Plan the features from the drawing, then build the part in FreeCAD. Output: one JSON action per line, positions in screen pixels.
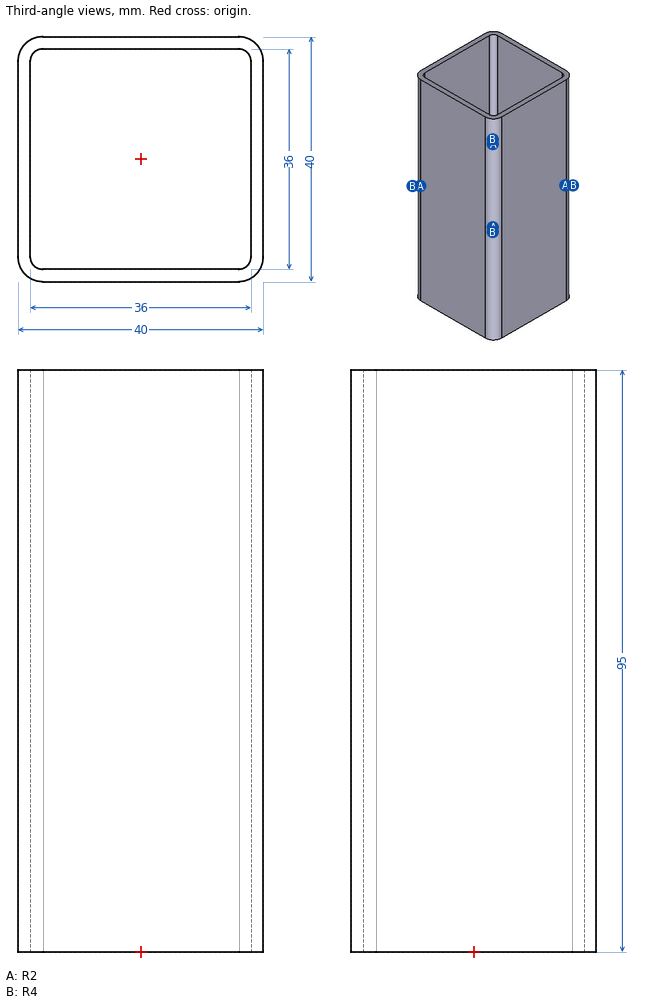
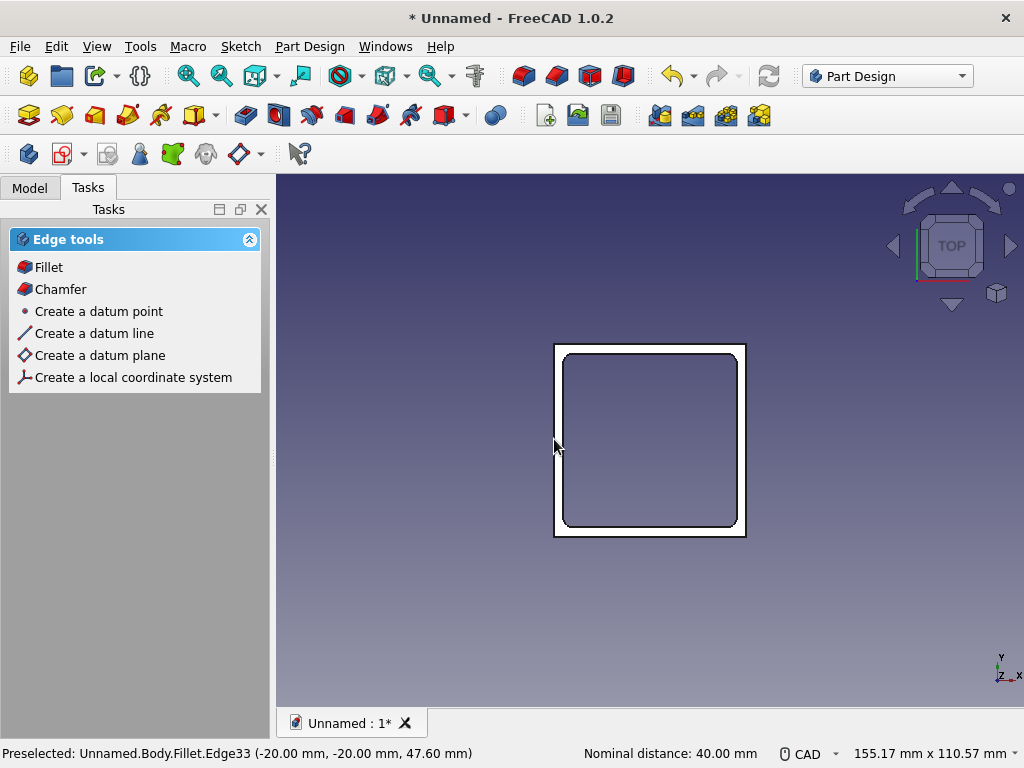
{"action": "key", "text": "v f"}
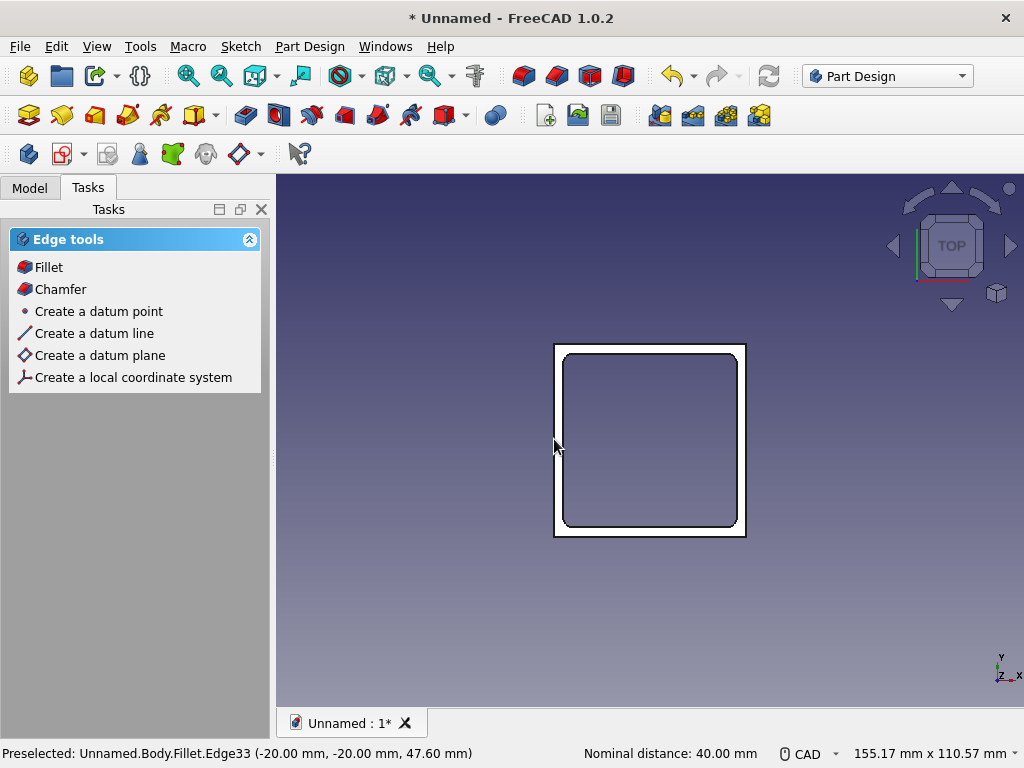
{"action": "key", "text": "1"}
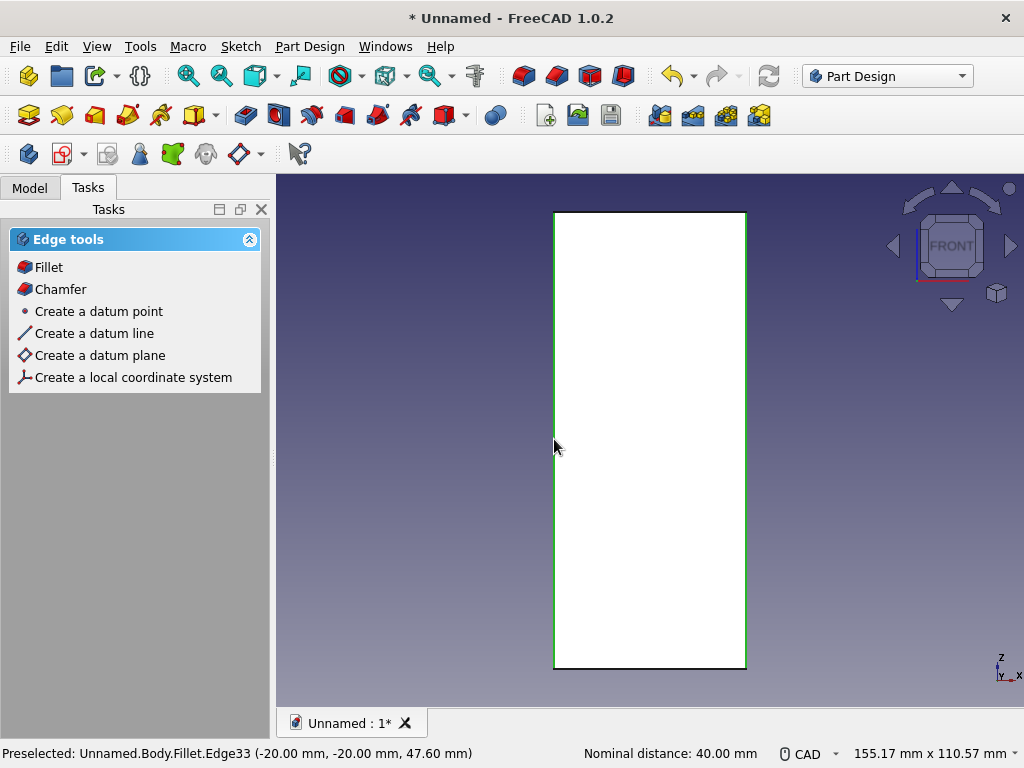
{"action": "key", "text": "3"}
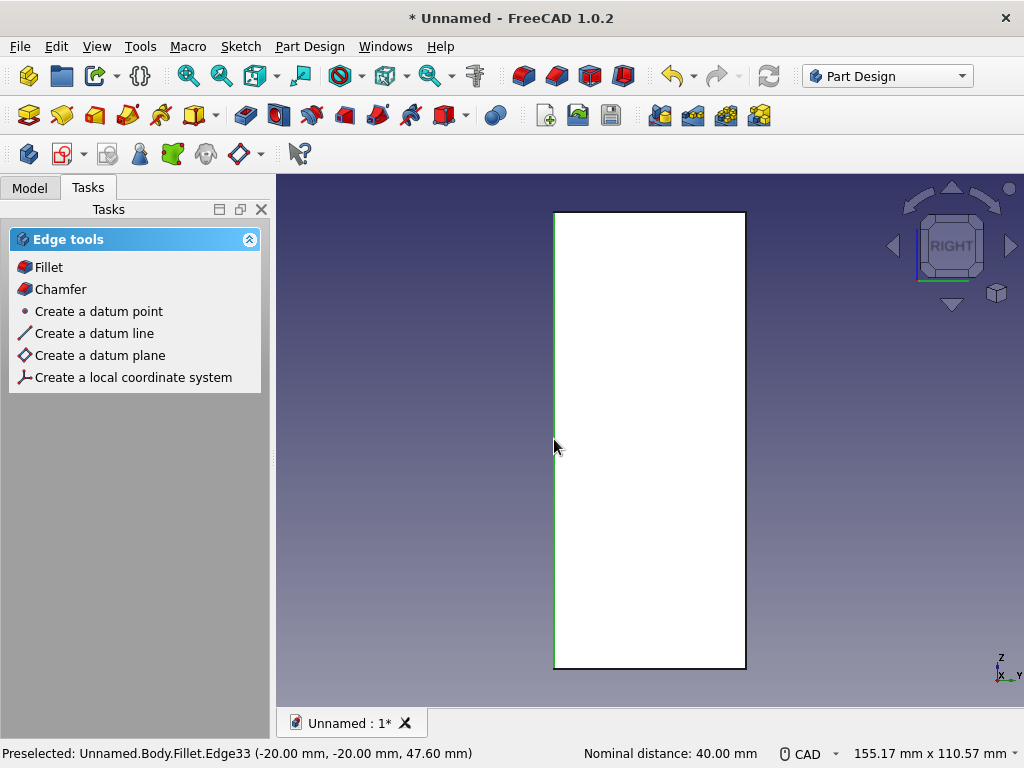
{"action": "left_click", "coordinate": [746, 439], "text": "ctrl"}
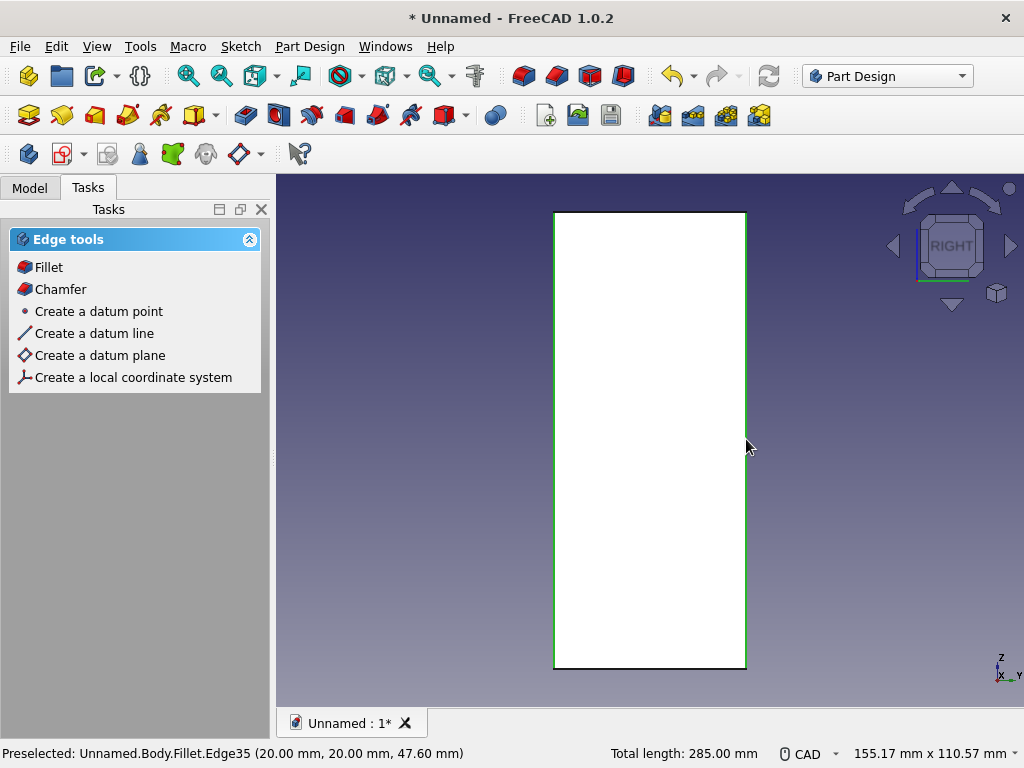
{"action": "key", "text": "5"}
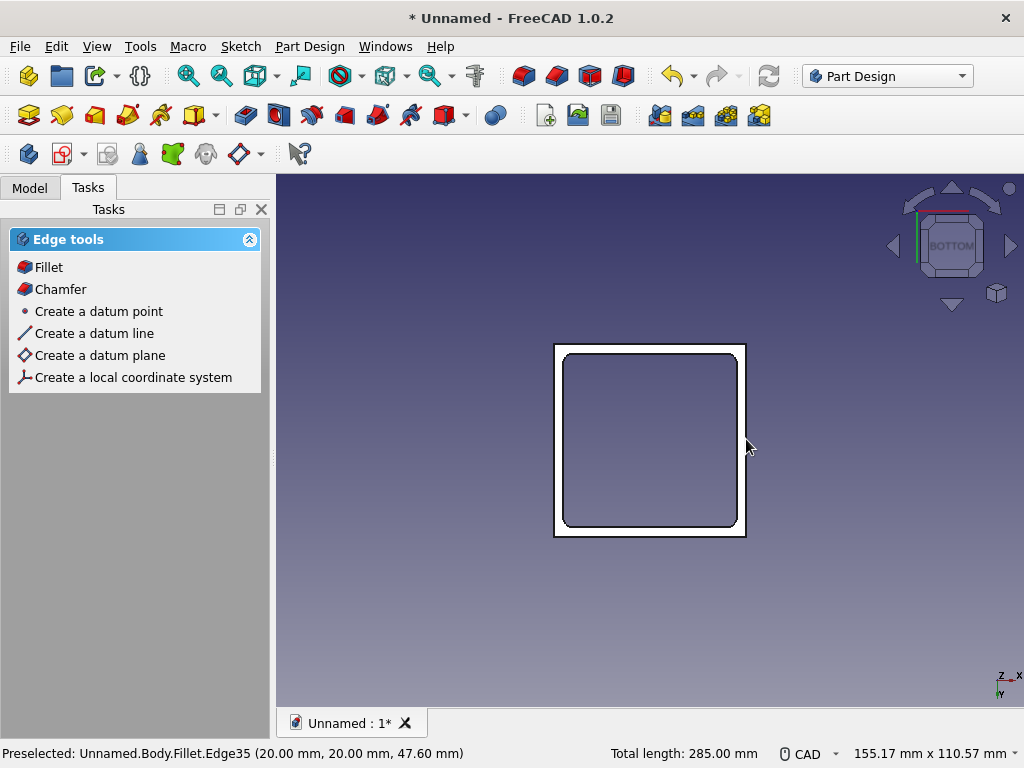
{"action": "left_click", "coordinate": [189, 76]}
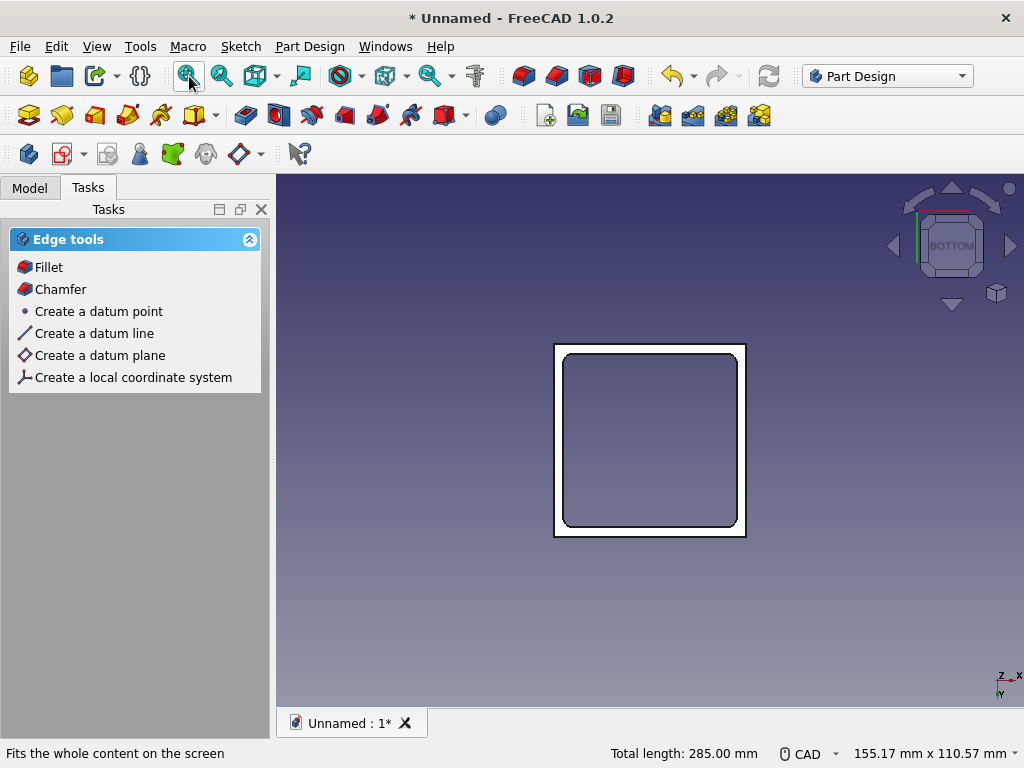
{"action": "key", "text": "4"}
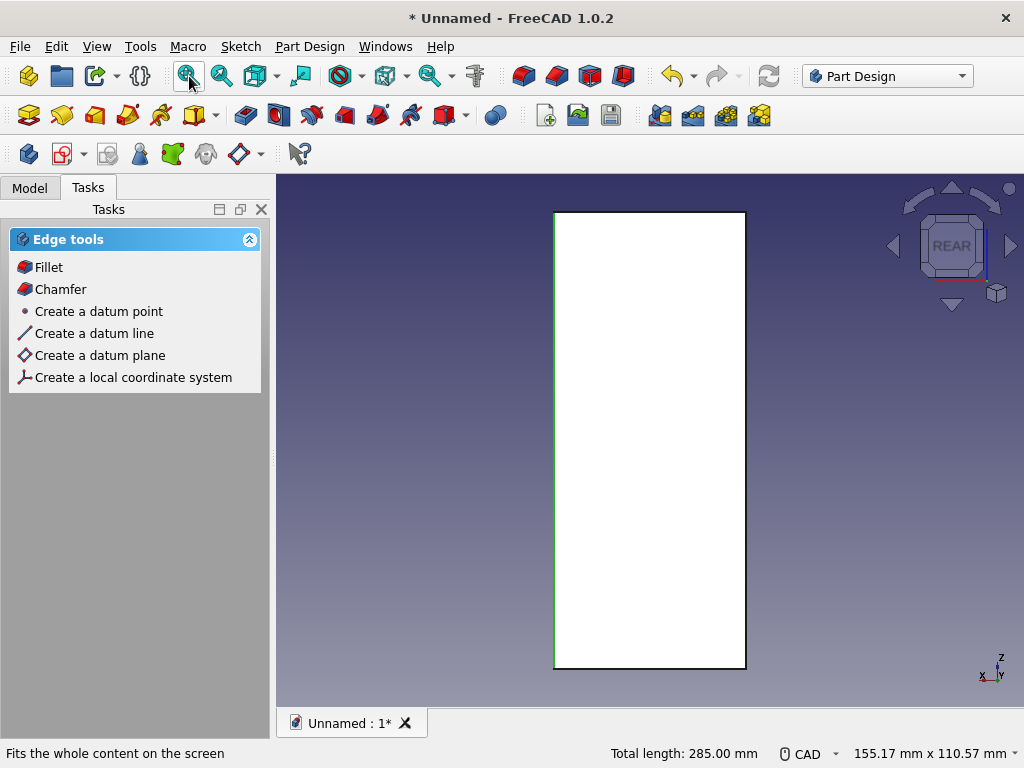
{"action": "left_click", "coordinate": [746, 440], "text": "ctrl"}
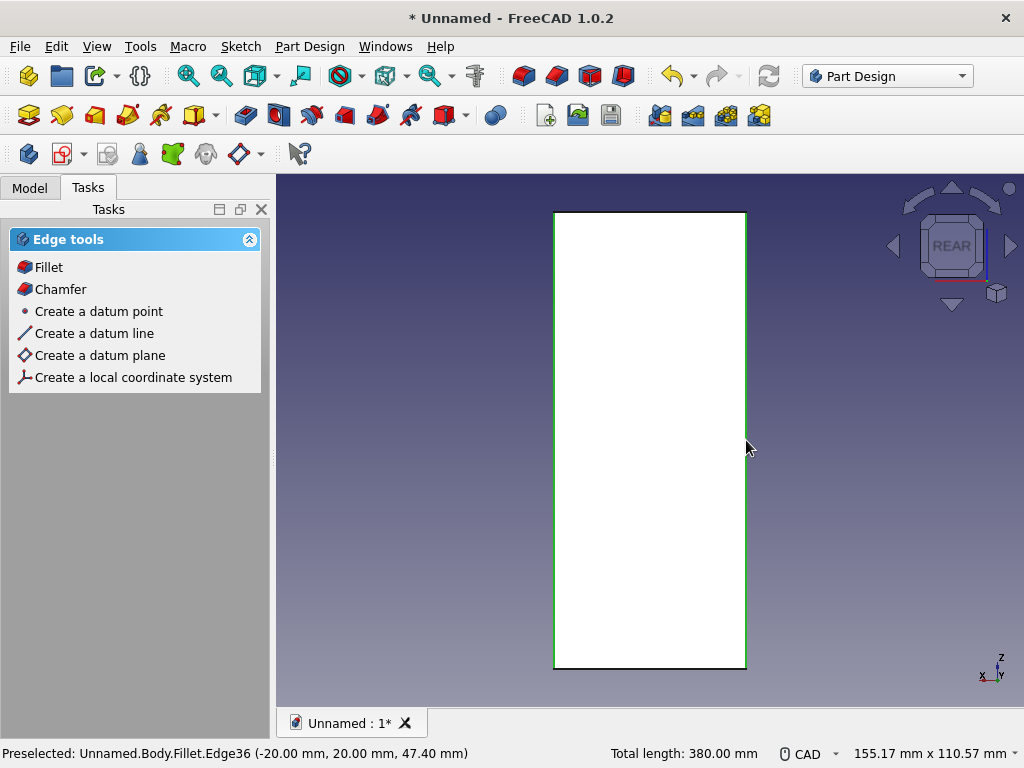
{"action": "left_click", "coordinate": [524, 76]}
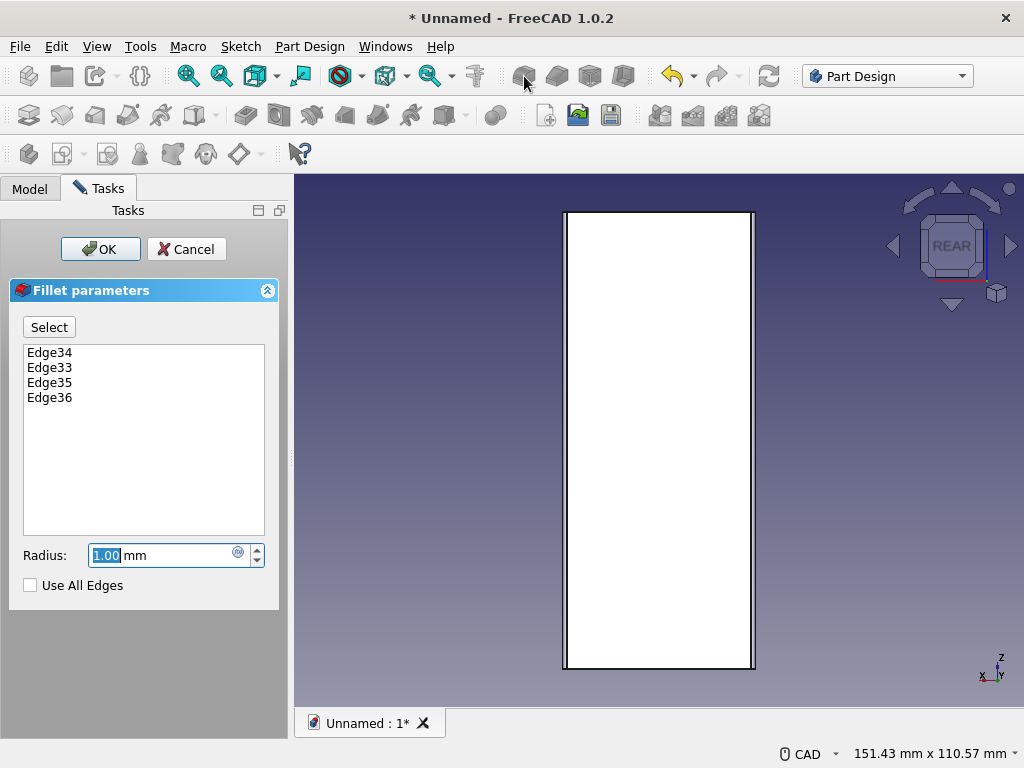
{"action": "type", "text": "4"}
{"action": "key", "text": "Tab"}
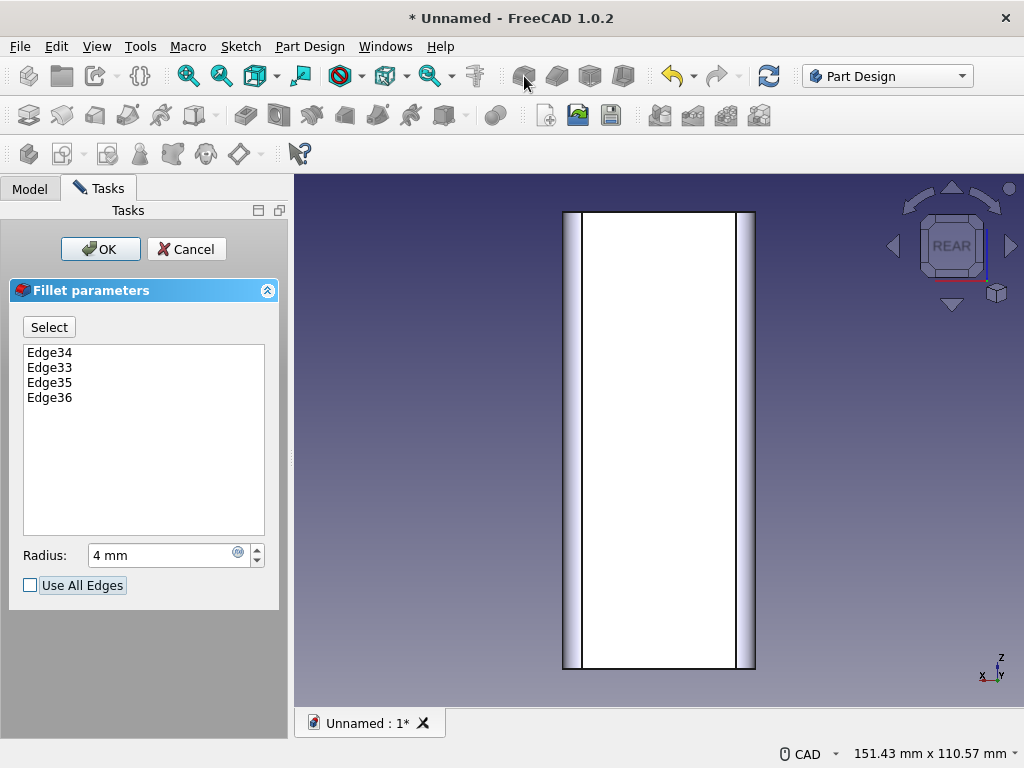
{"action": "left_click", "coordinate": [101, 249]}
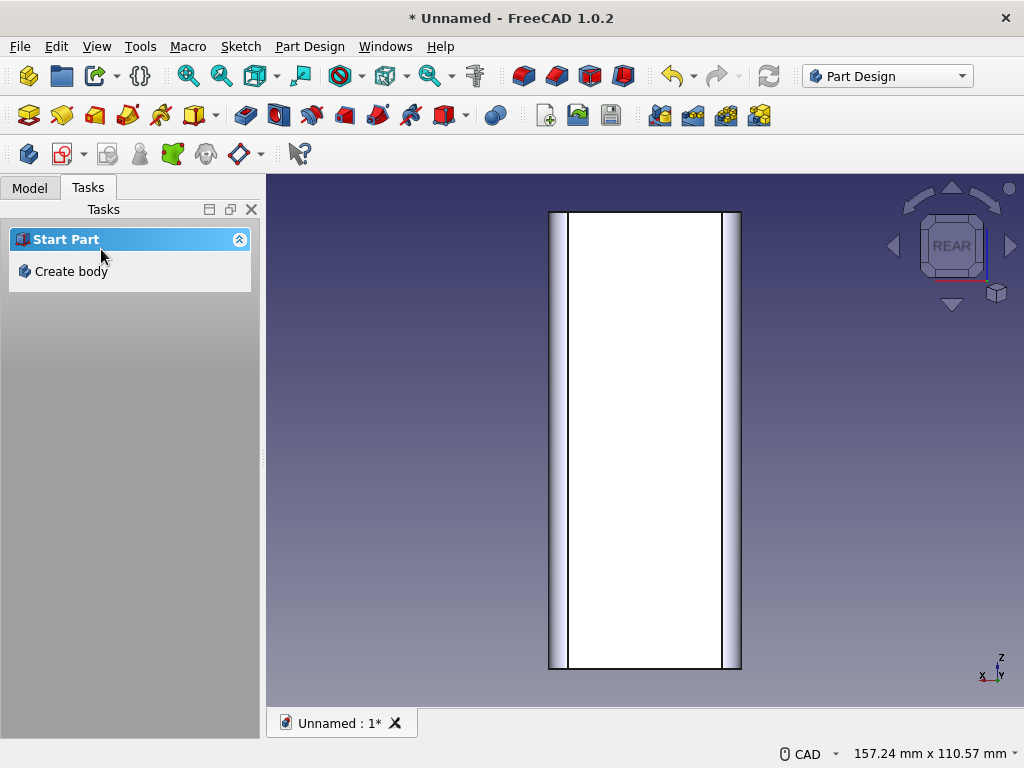
{"action": "key", "text": "0"}